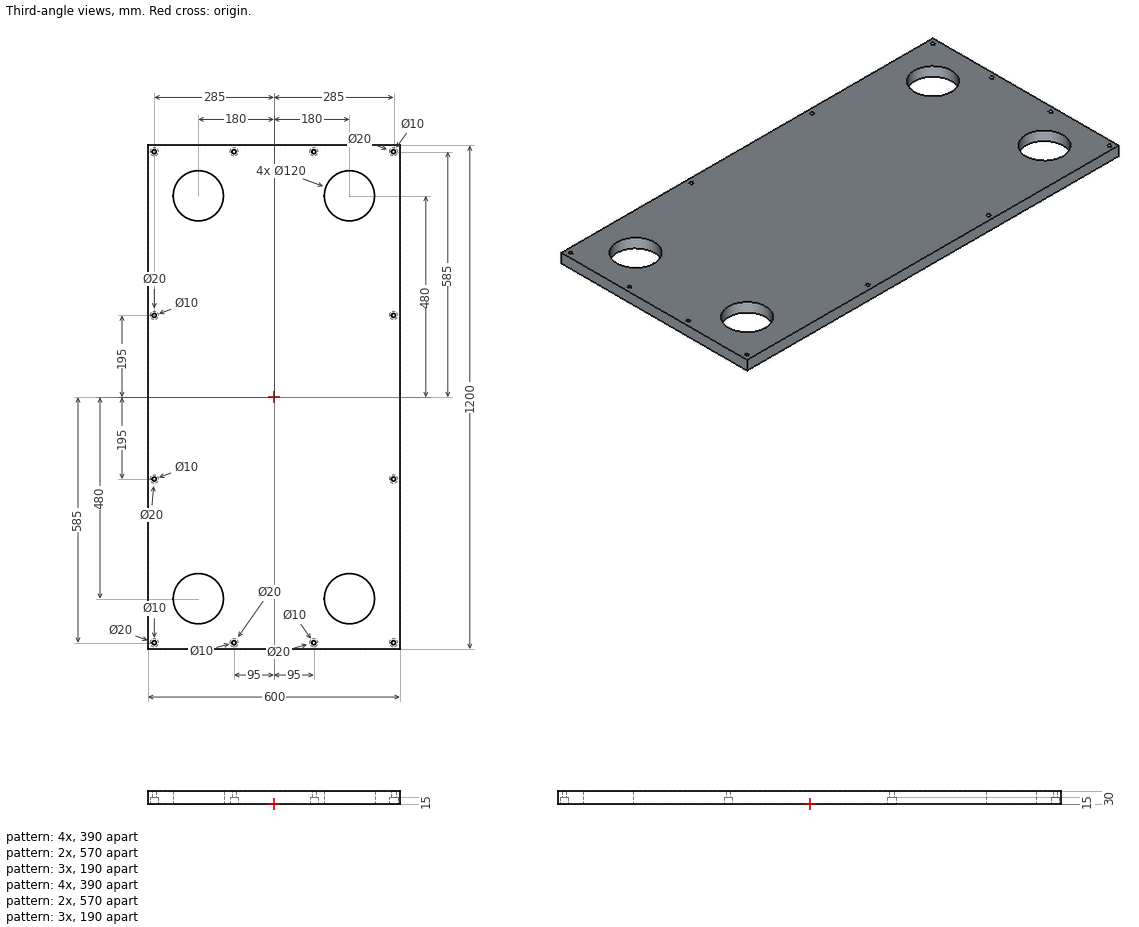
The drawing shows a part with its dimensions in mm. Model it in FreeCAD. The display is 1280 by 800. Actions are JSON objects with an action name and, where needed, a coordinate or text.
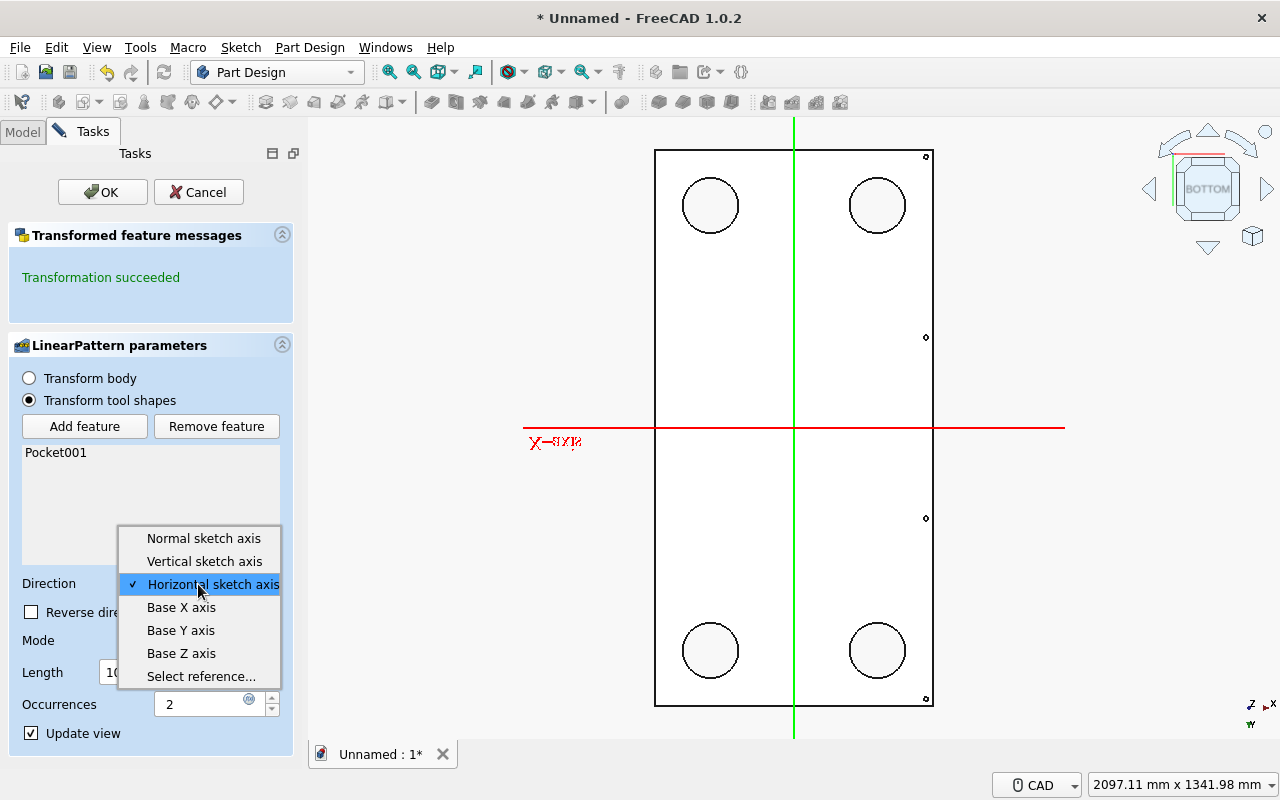
{"action": "left_click", "coordinate": [198, 608]}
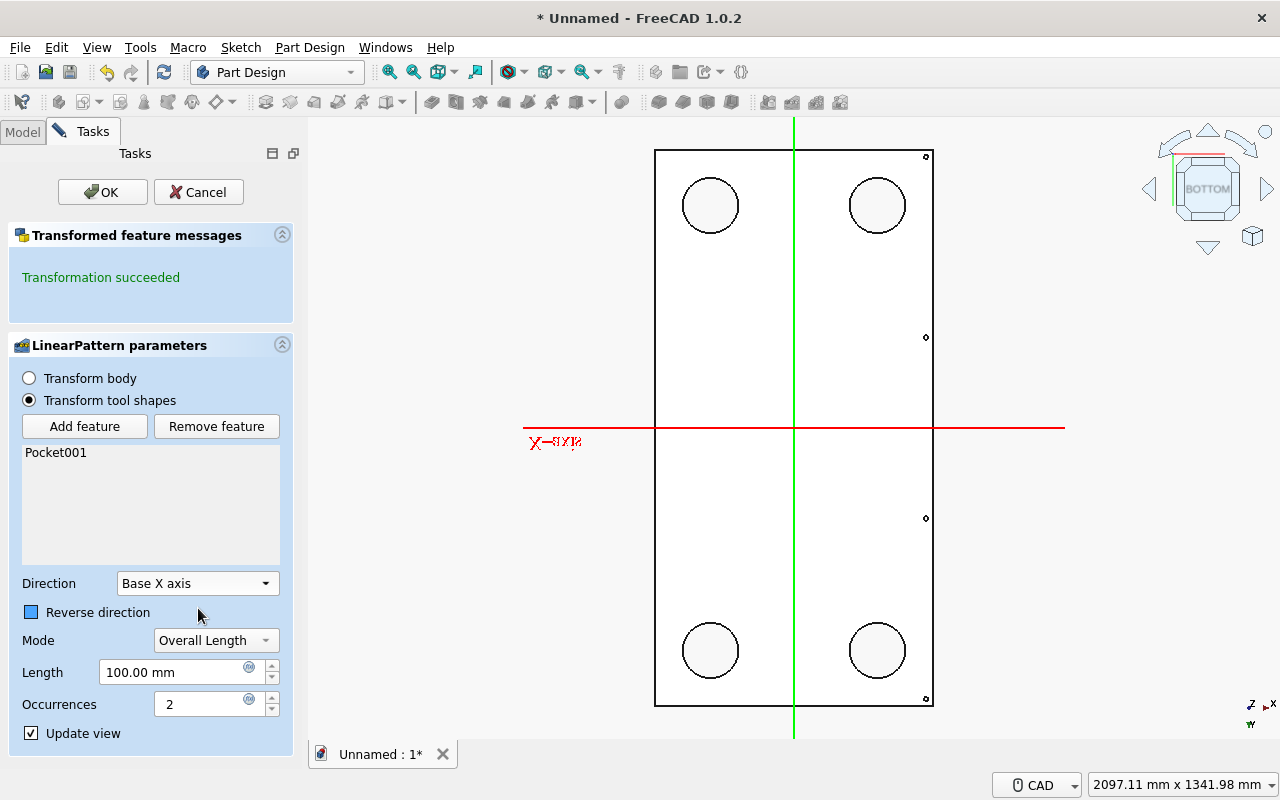
{"action": "left_click", "coordinate": [217, 640]}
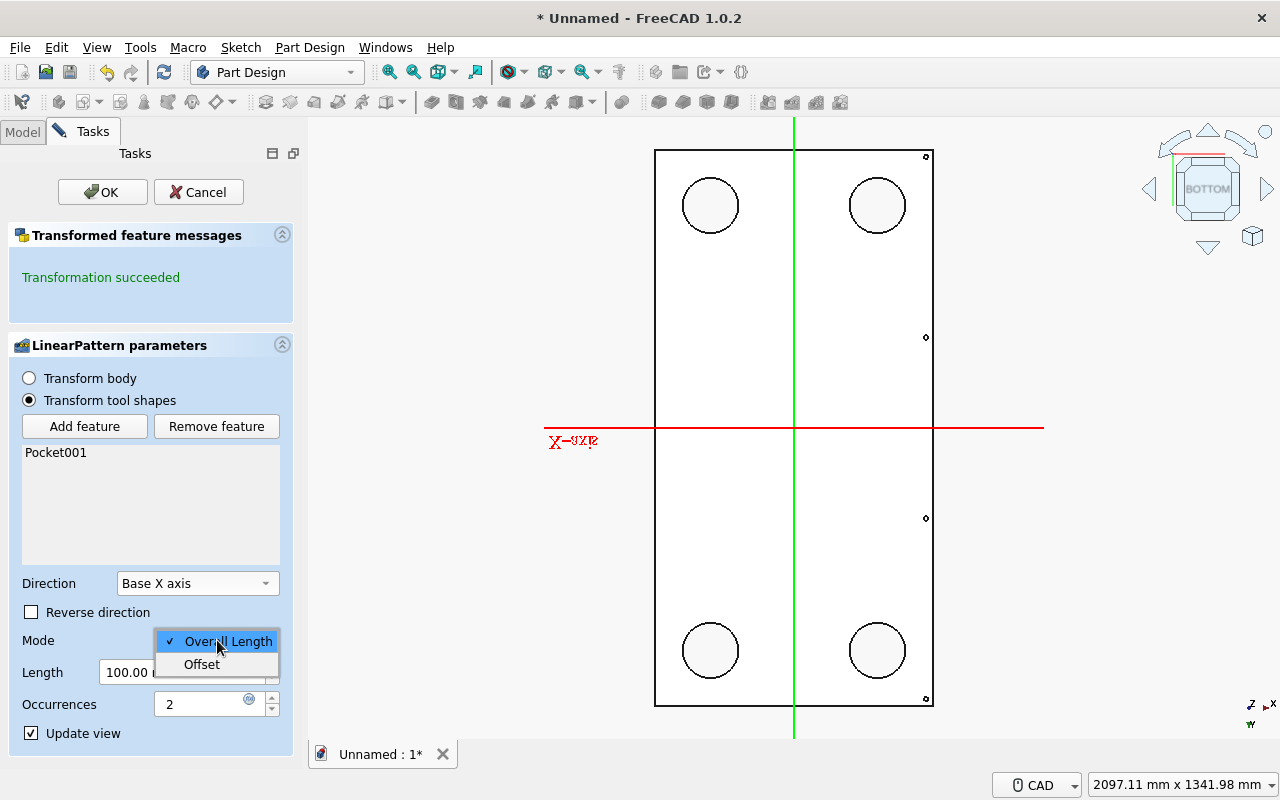
{"action": "left_click", "coordinate": [216, 664]}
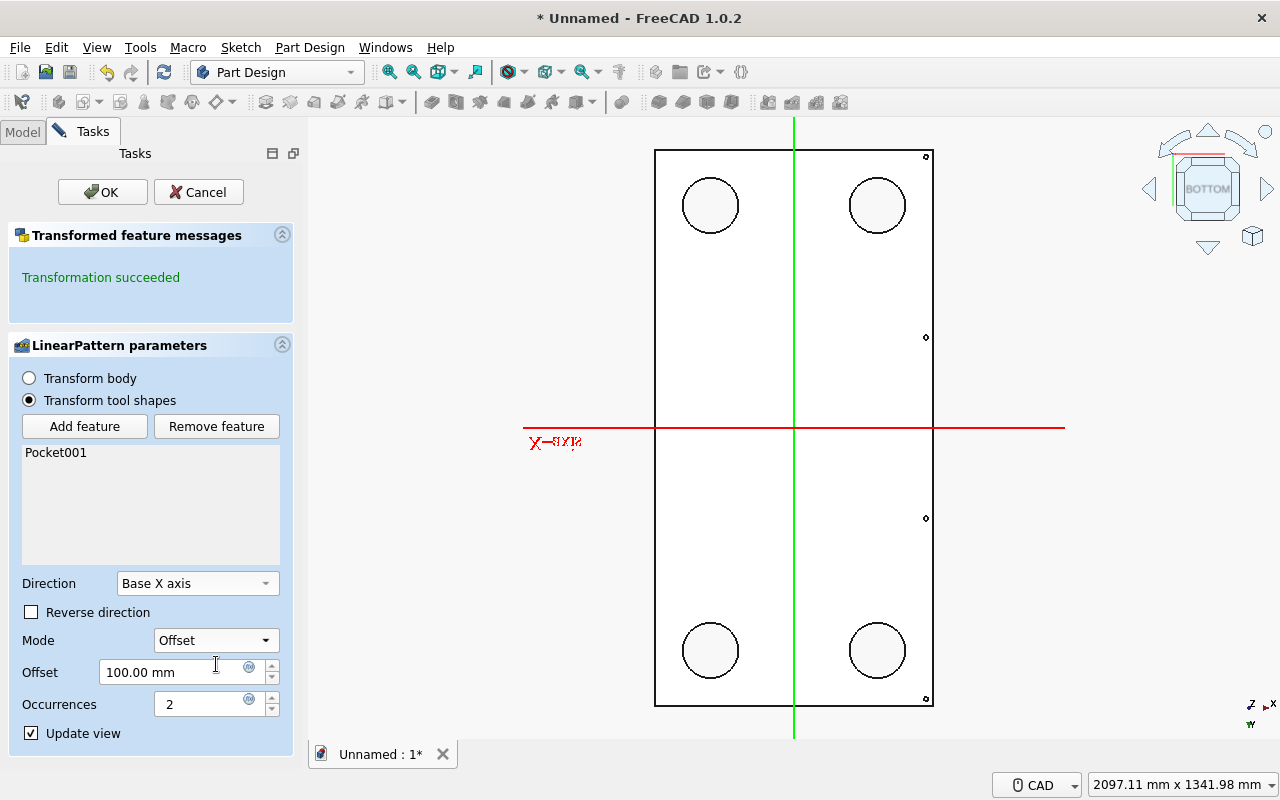
{"action": "triple_click", "coordinate": [182, 672]}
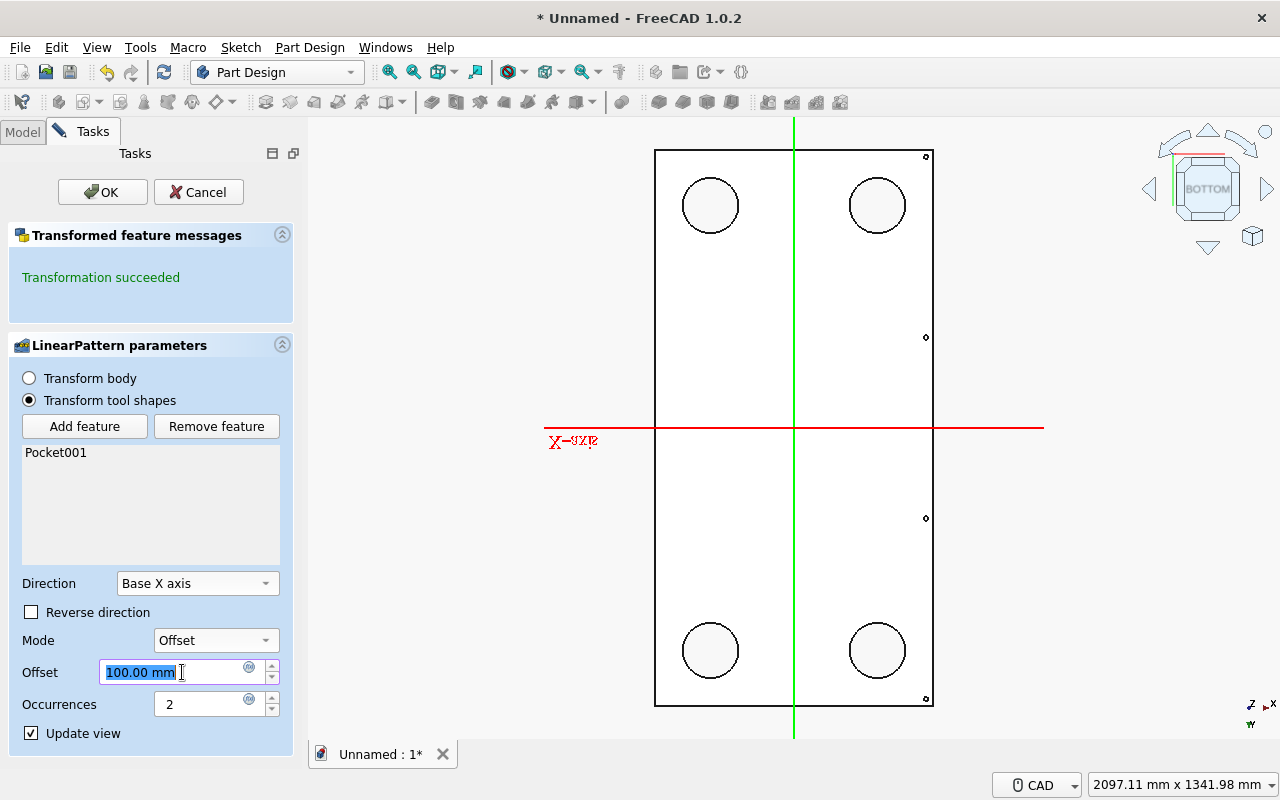
{"action": "type", "text": "570"}
{"action": "key", "text": "Tab"}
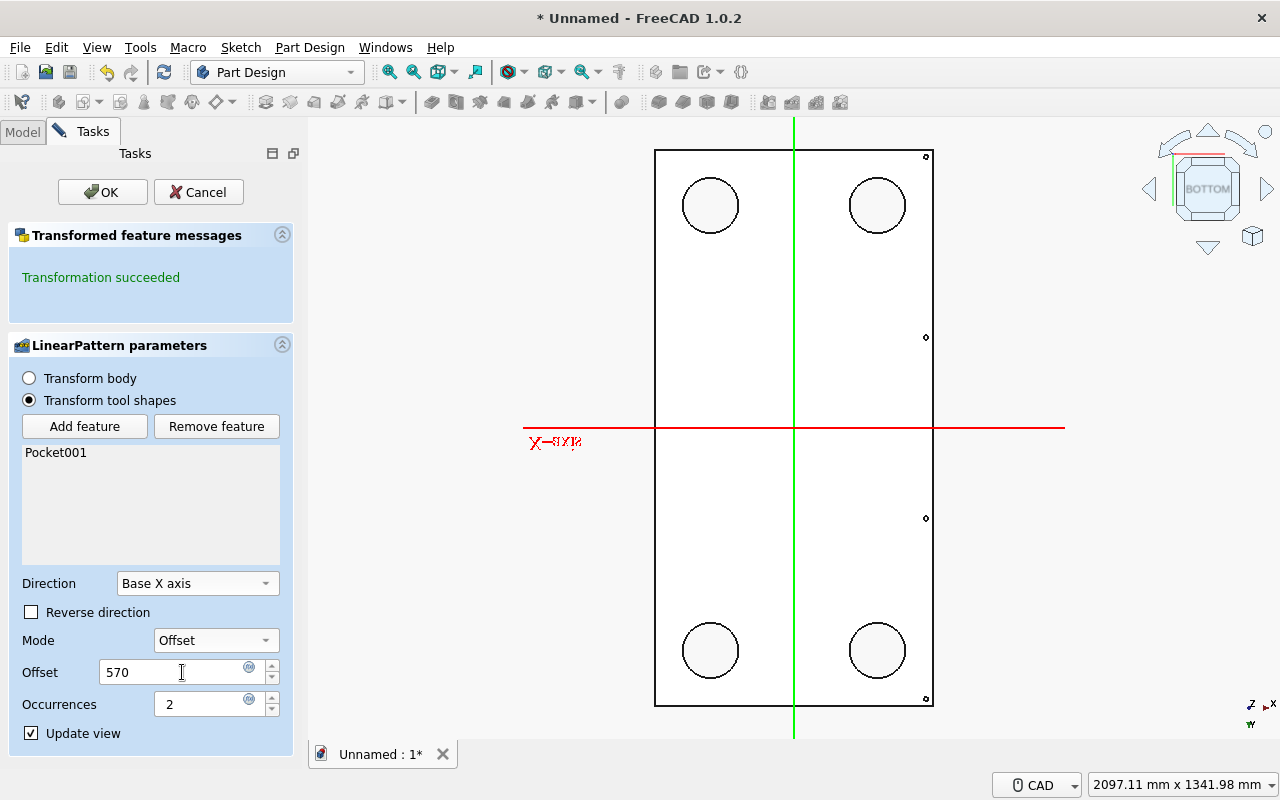
{"action": "triple_click", "coordinate": [209, 704]}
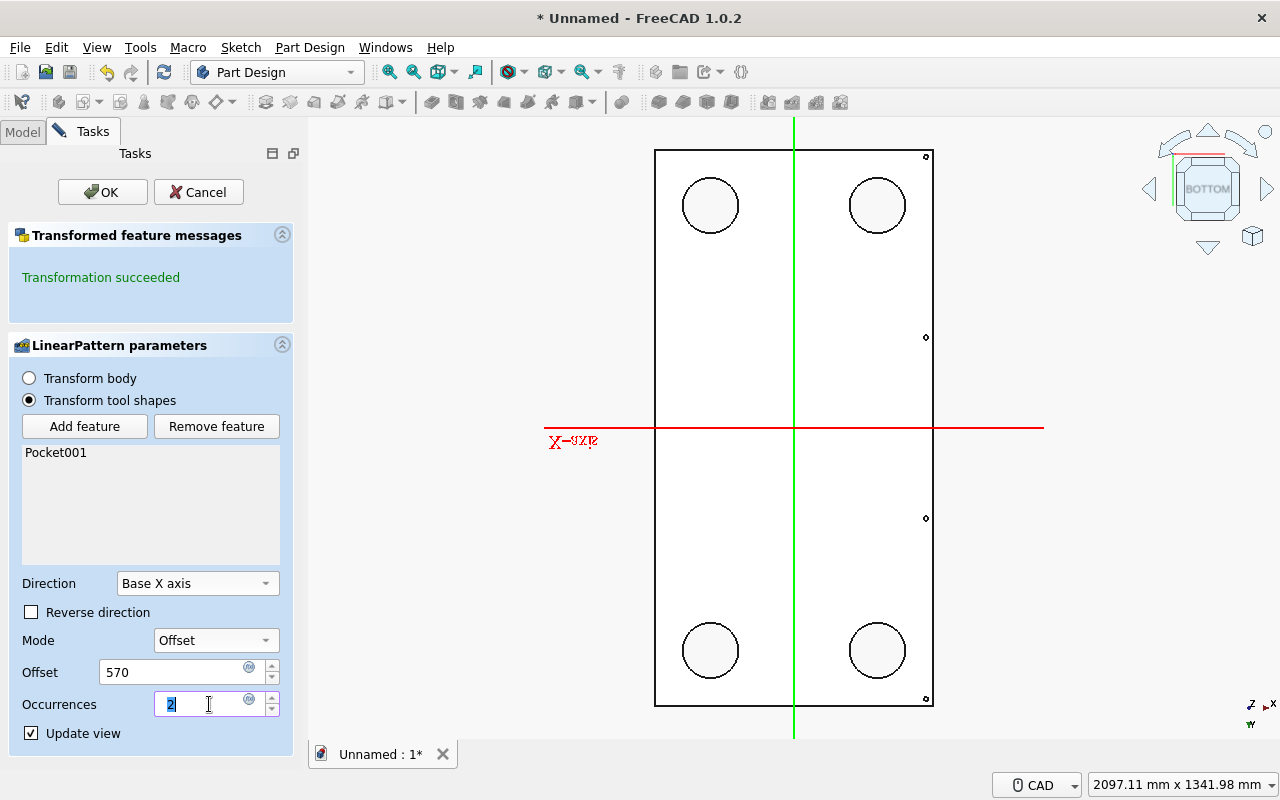
{"action": "type", "text": "2"}
{"action": "key", "text": "Tab"}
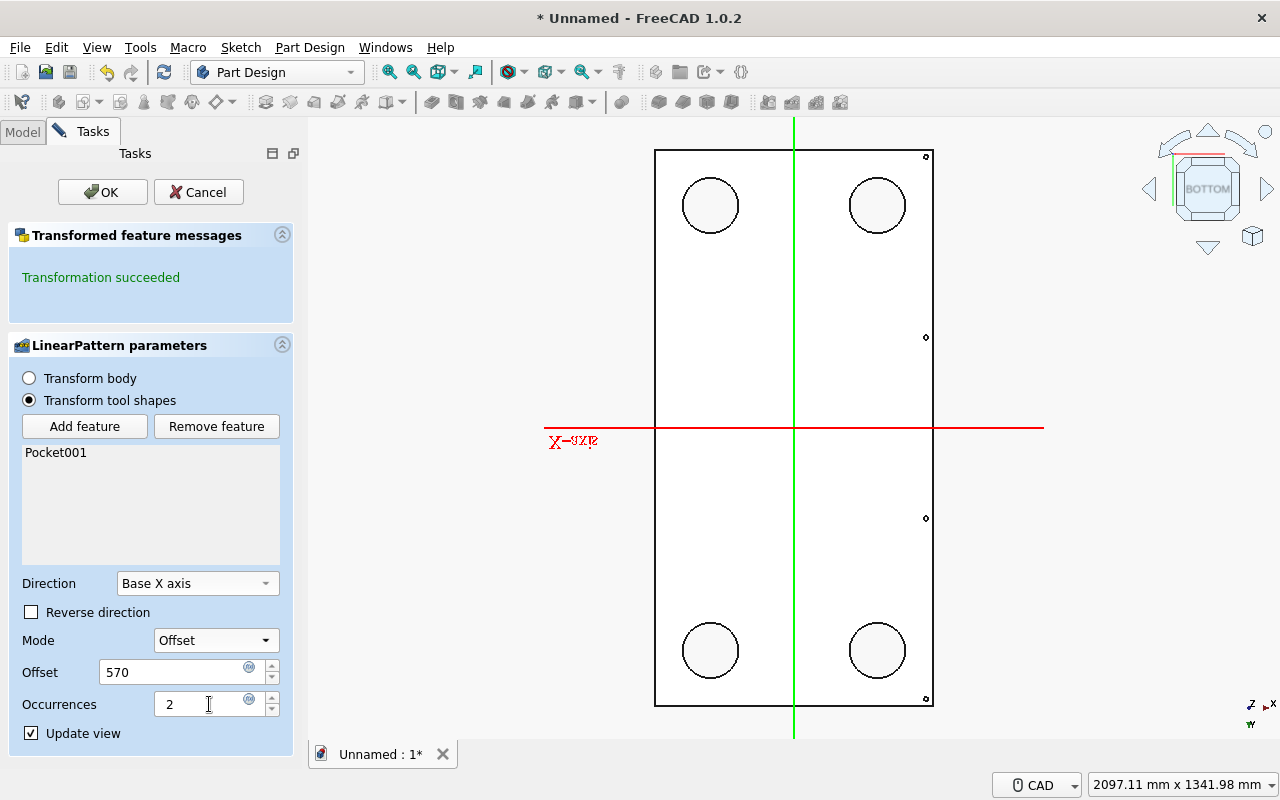
{"action": "left_click", "coordinate": [30, 612]}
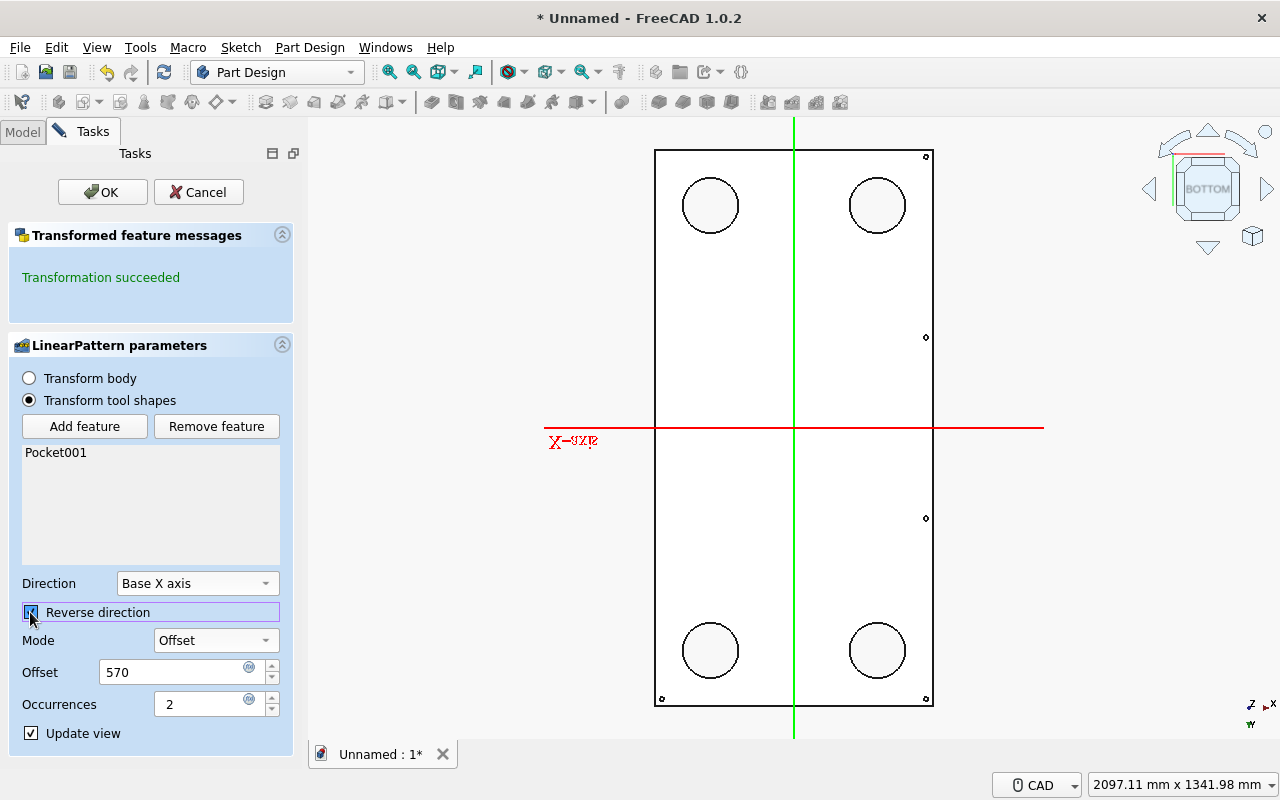
{"action": "left_click", "coordinate": [103, 192]}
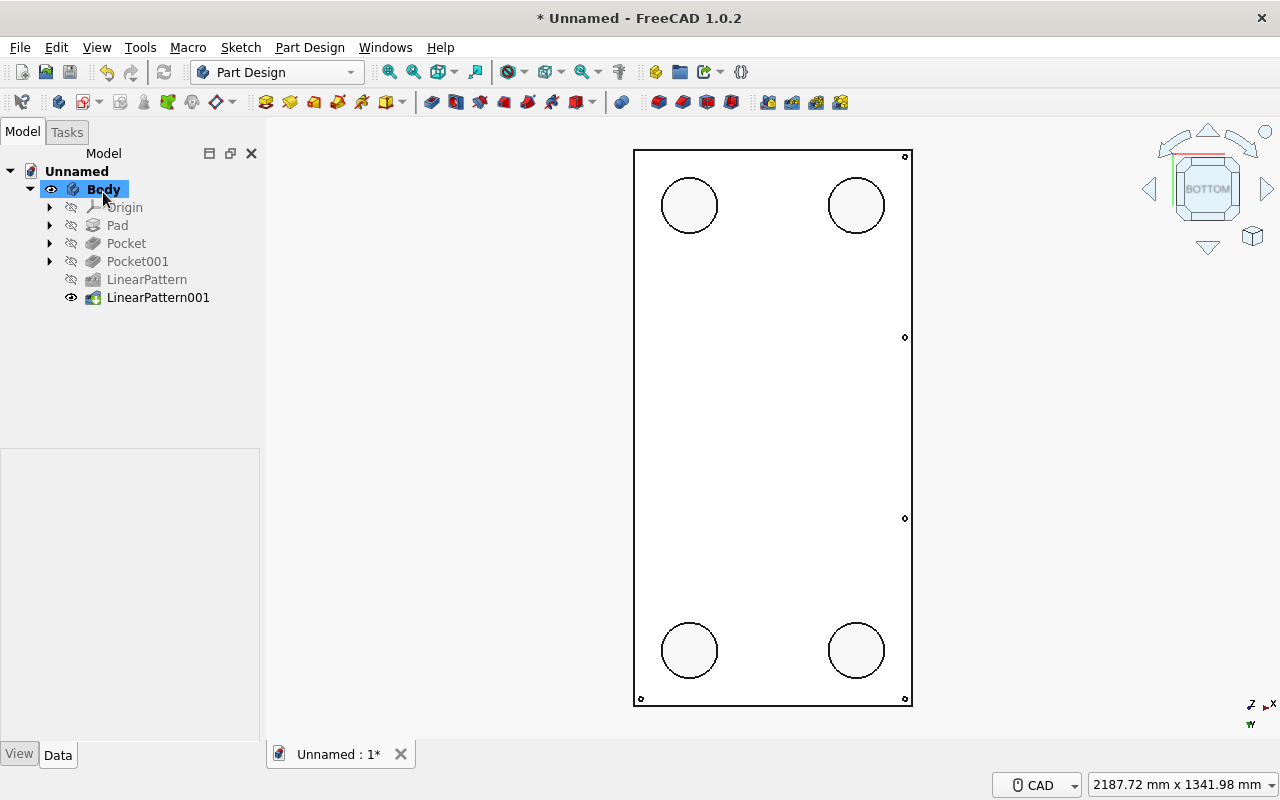
{"action": "left_click", "coordinate": [84, 102]}